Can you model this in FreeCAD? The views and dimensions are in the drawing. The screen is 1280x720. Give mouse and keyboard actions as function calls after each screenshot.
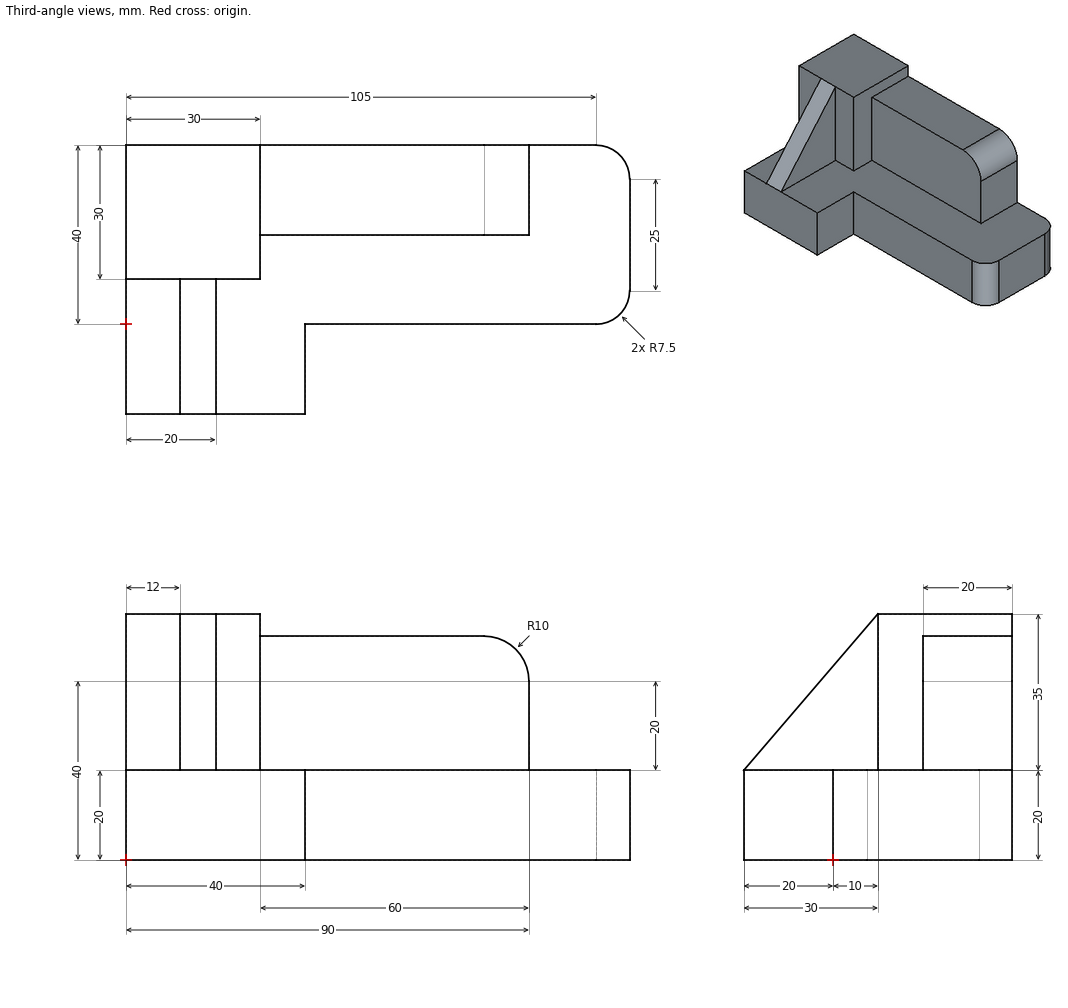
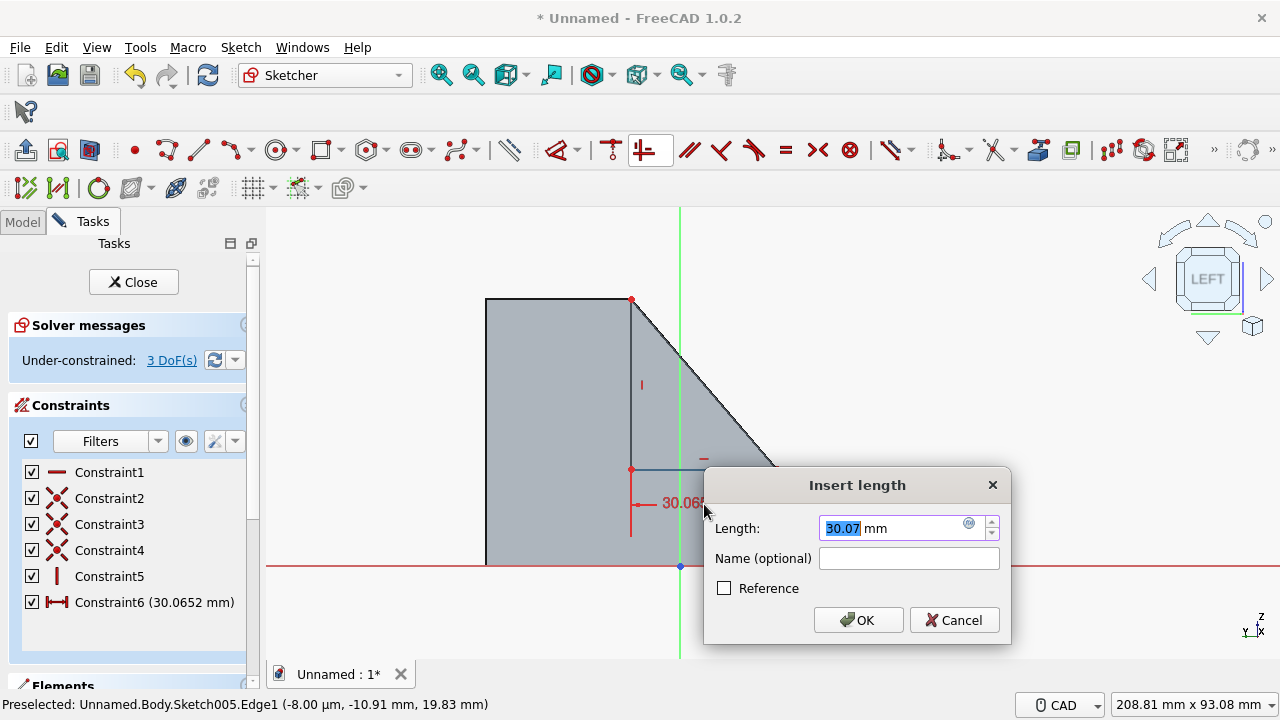
text(30)
key(Return)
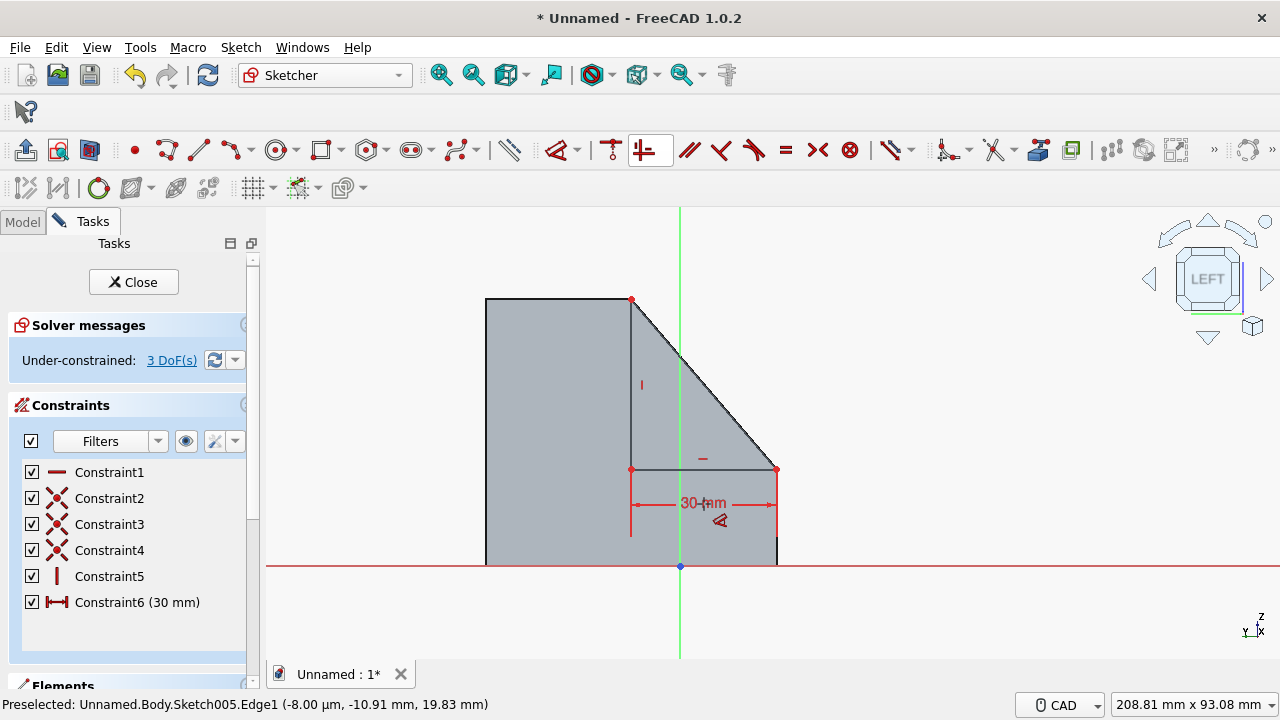
click(631, 351)
click(597, 385)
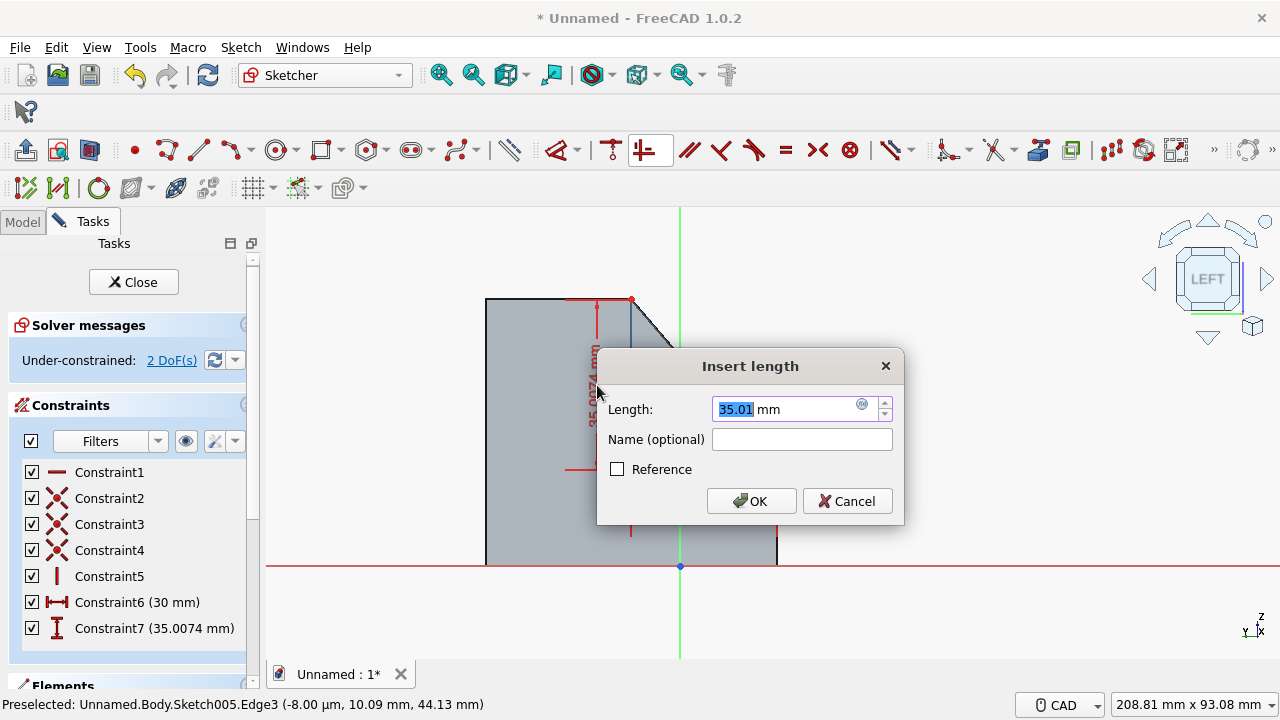
text(35)
key(Return)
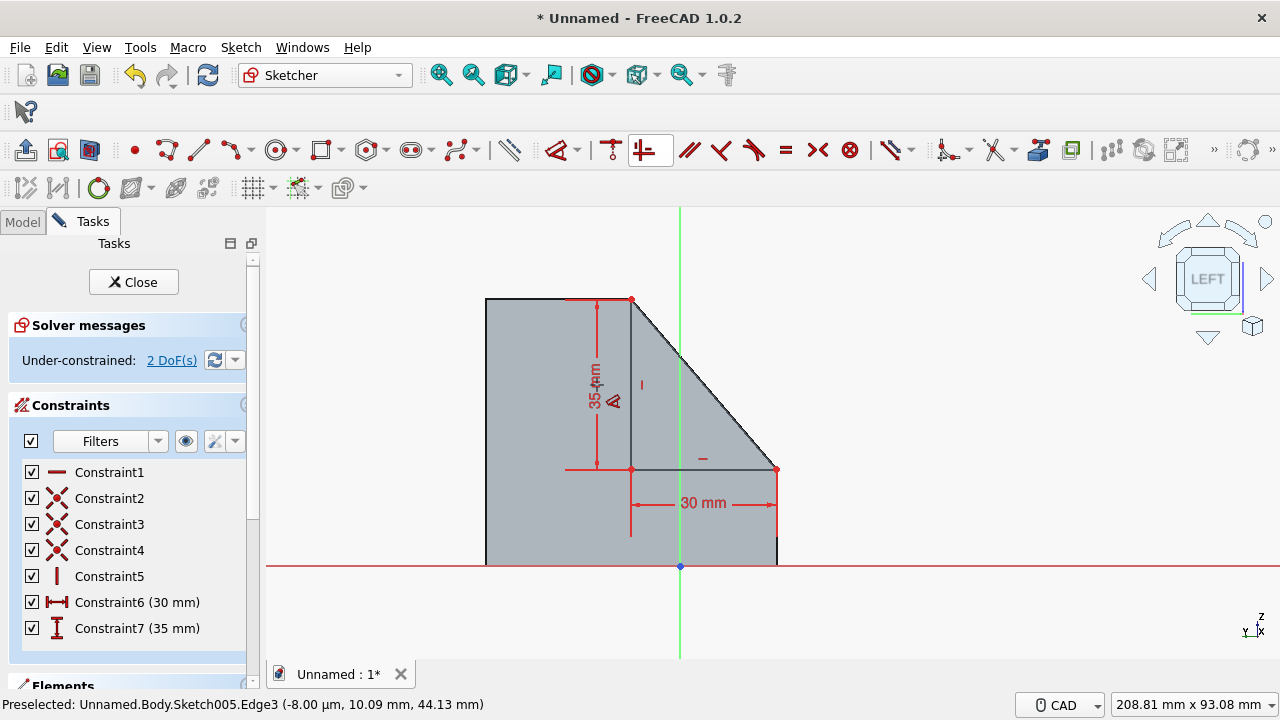
click(631, 470)
click(656, 600)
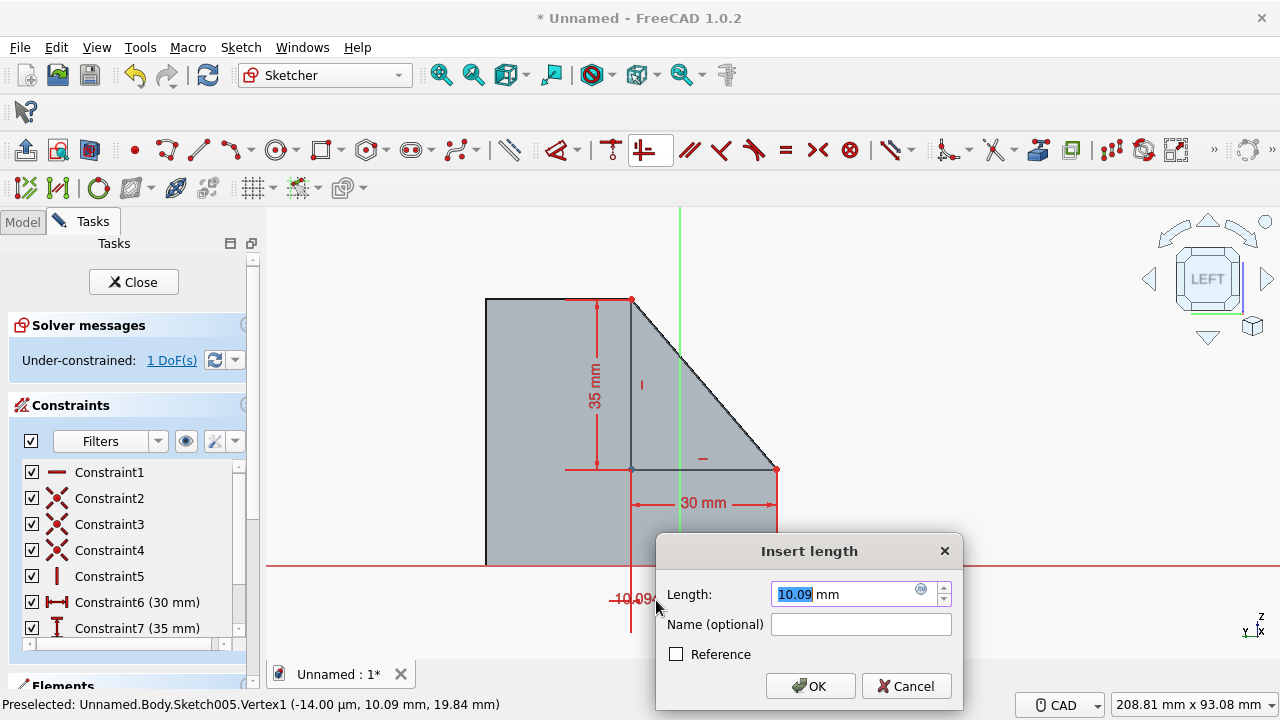
text(10)
key(Return)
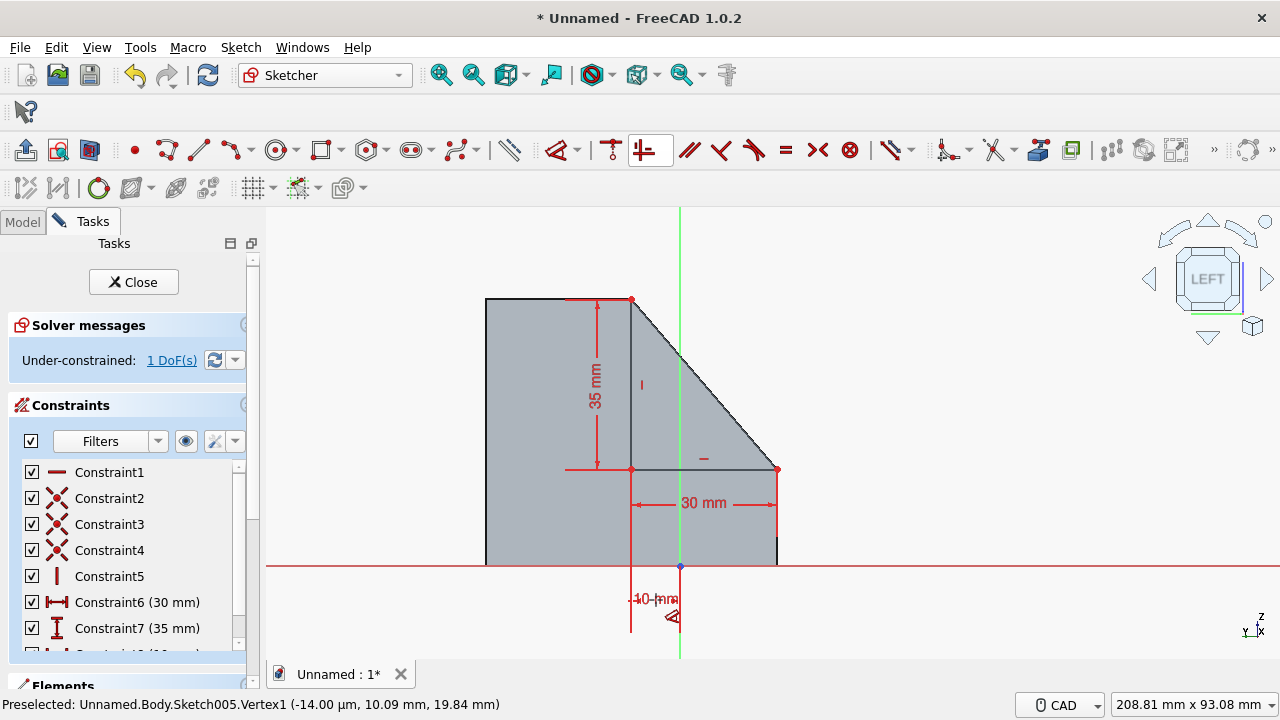
click(631, 470)
click(597, 518)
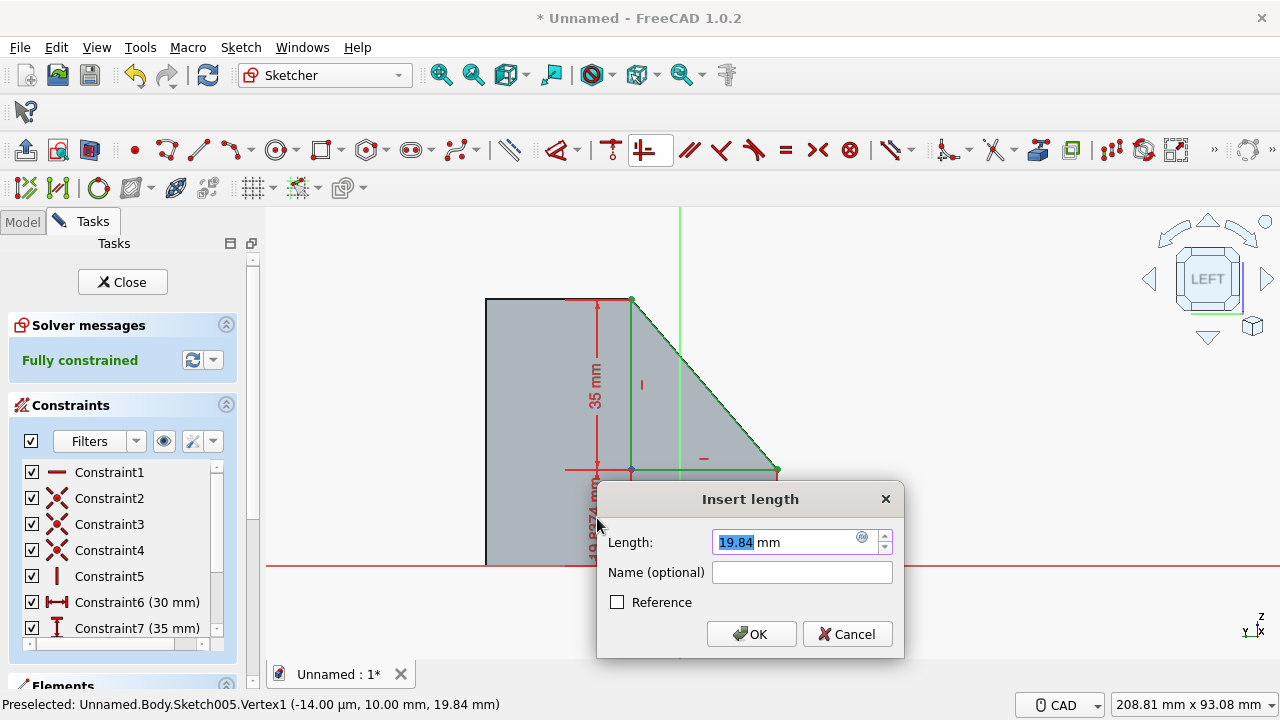
text(20)
key(Return)
key(Escape)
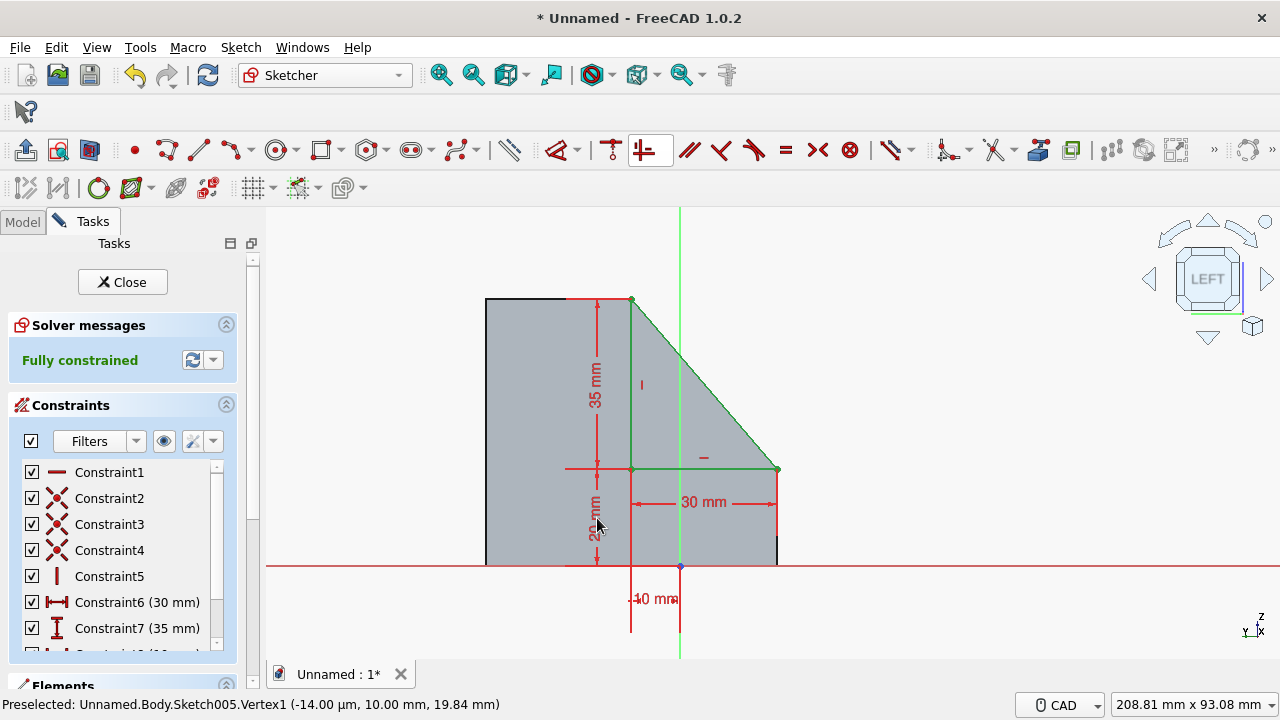
click(123, 282)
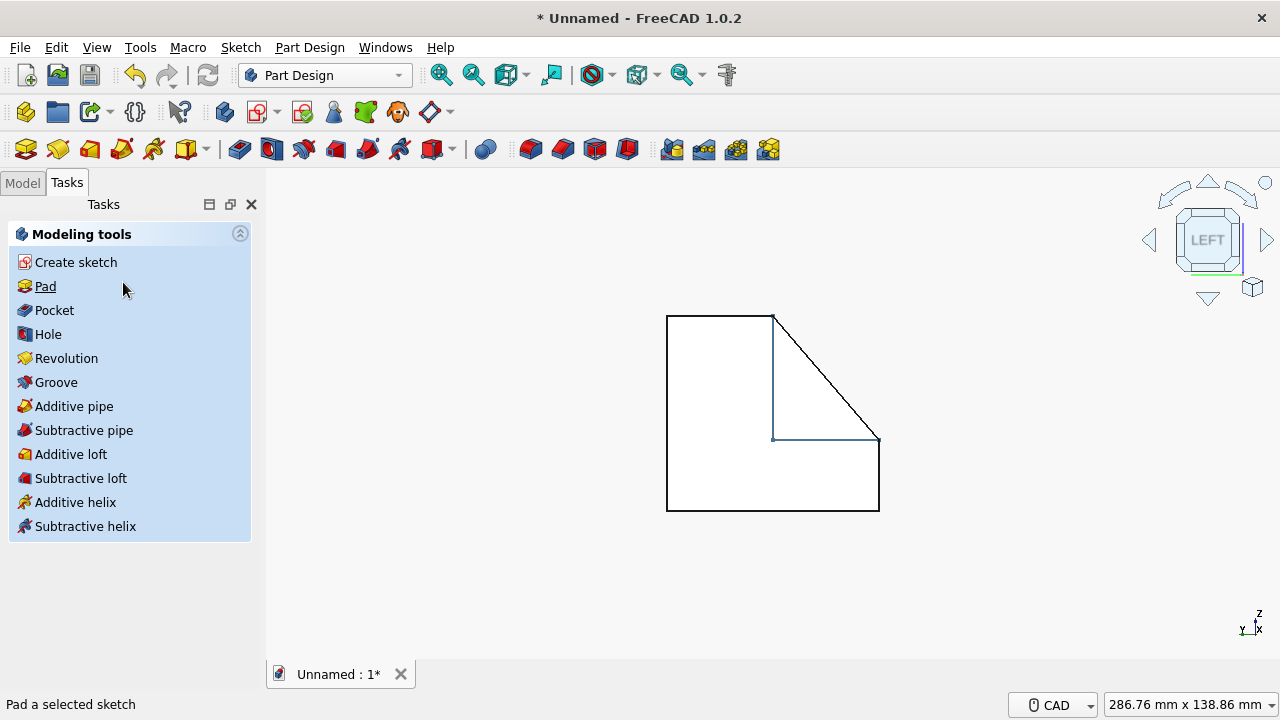
click(240, 150)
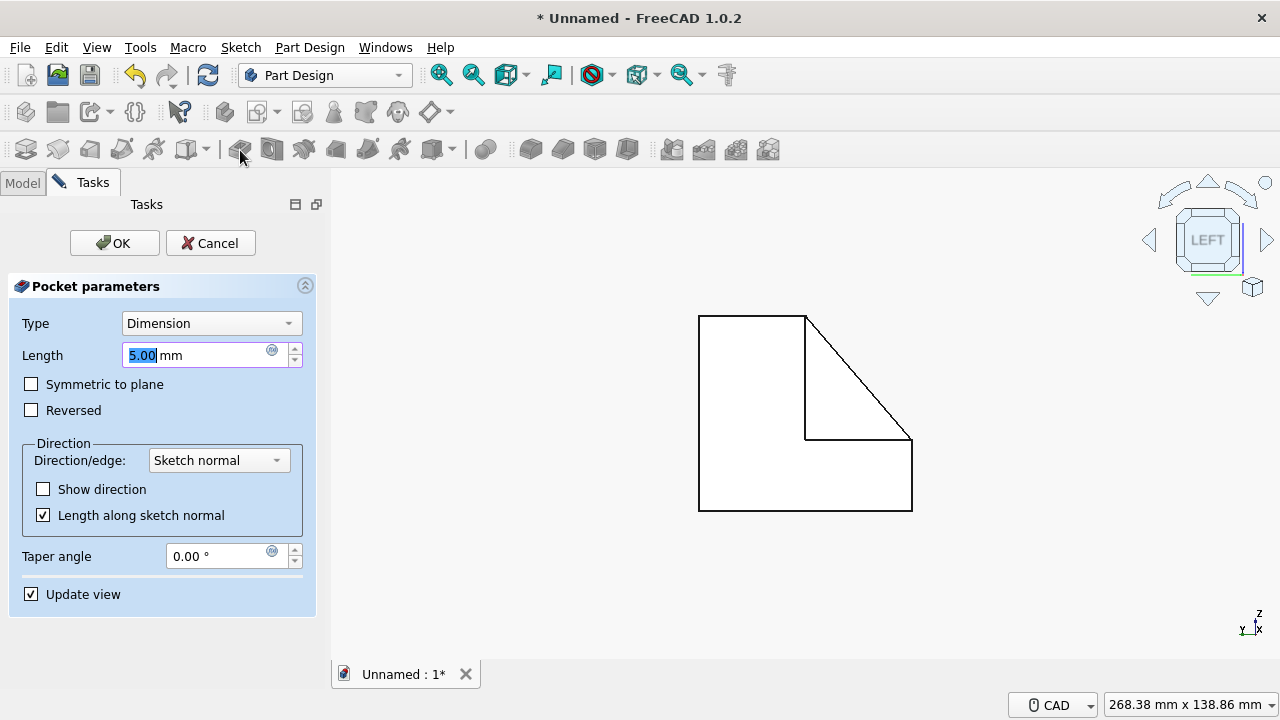
text(12)
key(Tab)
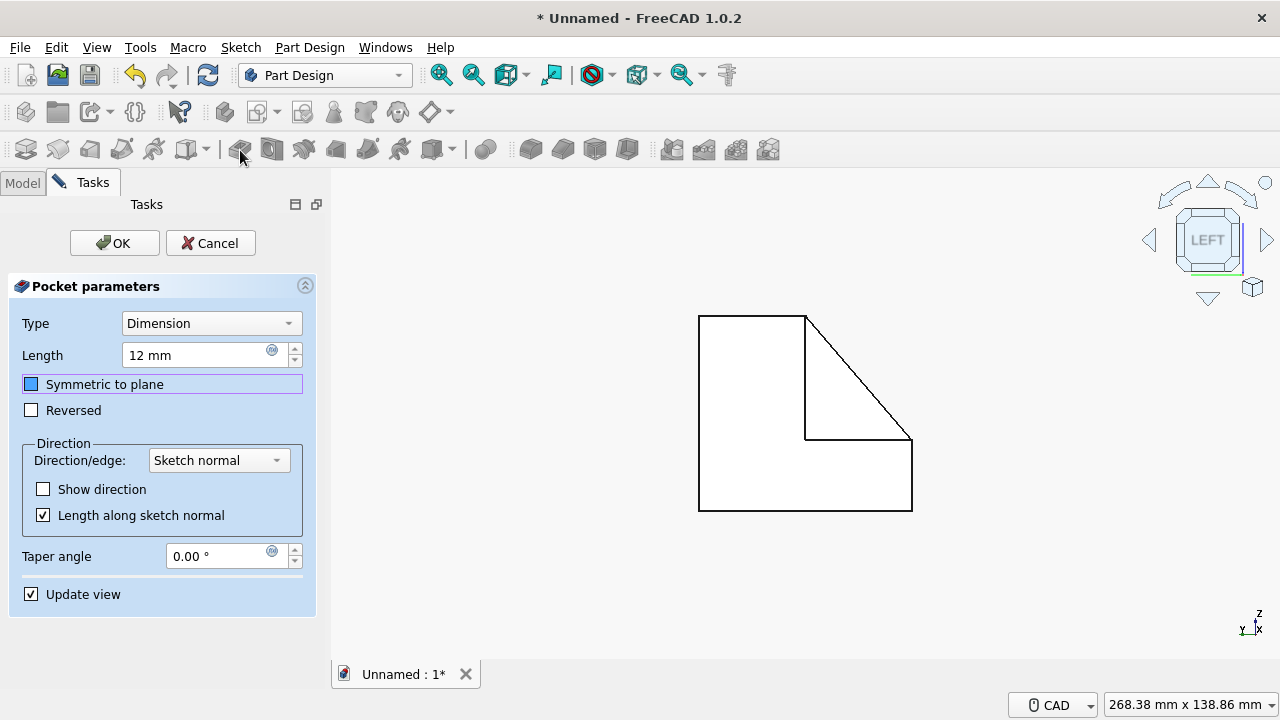
click(115, 243)